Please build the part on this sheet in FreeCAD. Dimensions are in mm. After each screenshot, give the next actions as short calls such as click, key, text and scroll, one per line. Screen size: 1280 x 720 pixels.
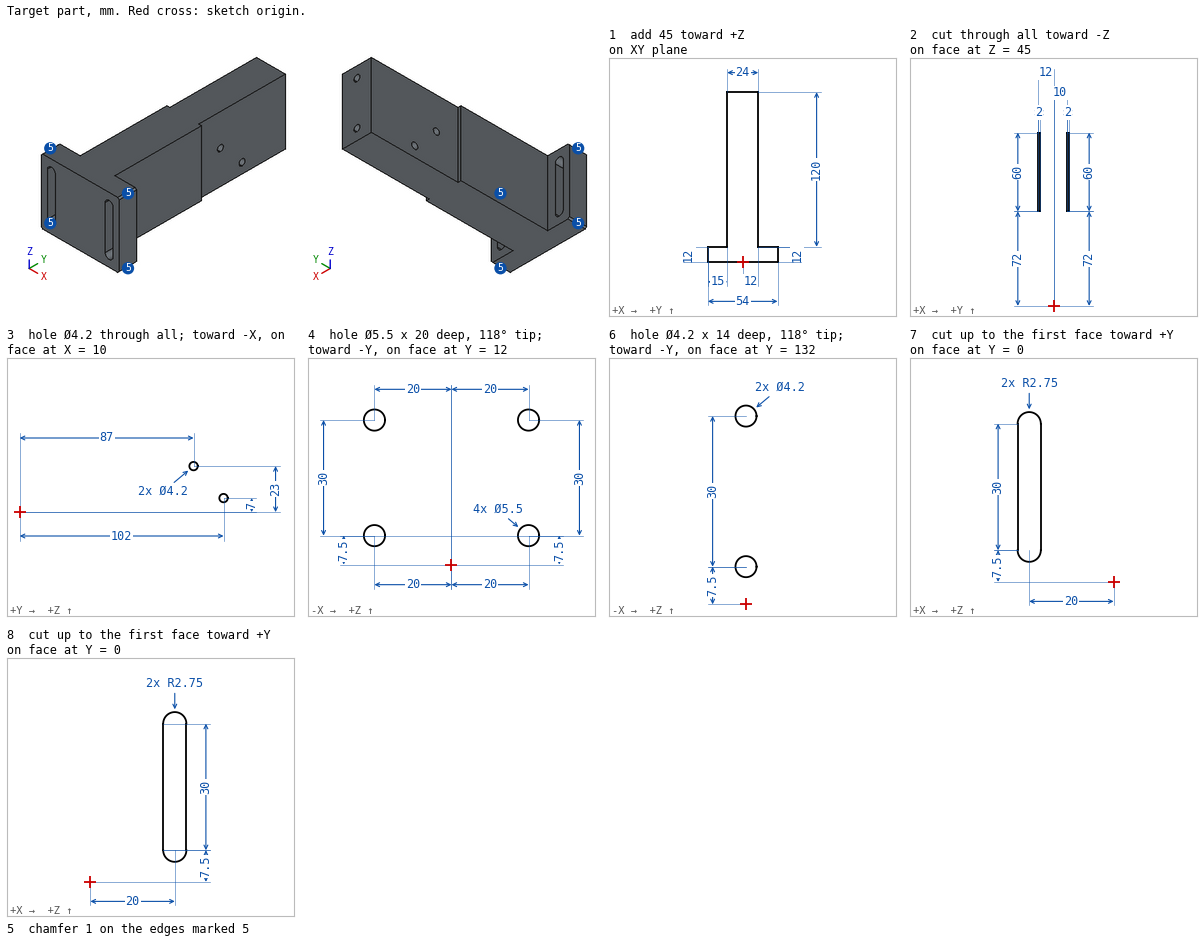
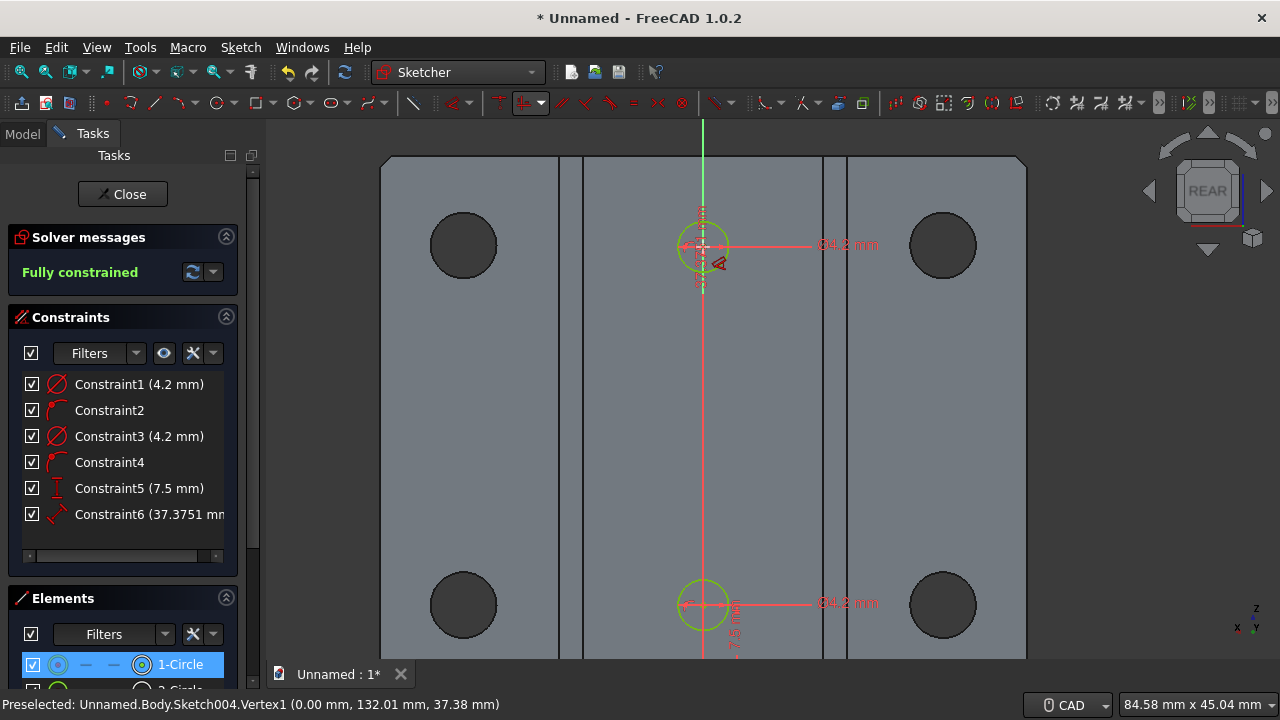
click(703, 605)
click(737, 426)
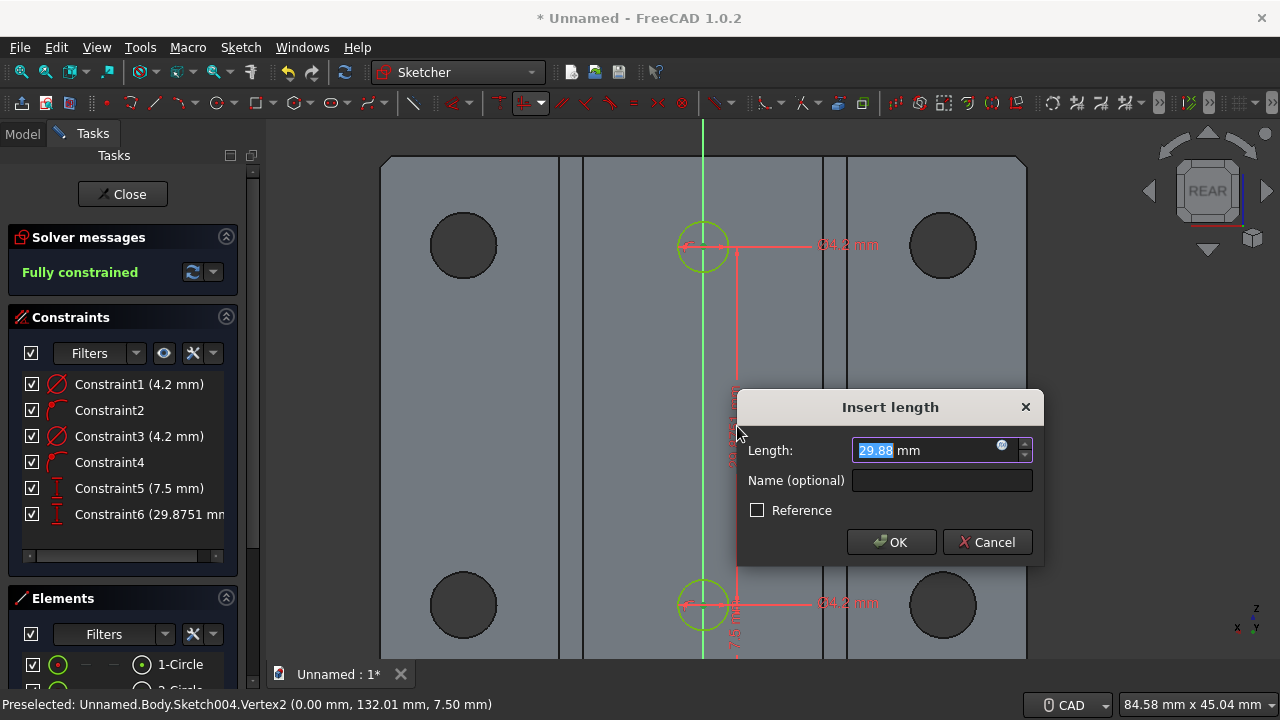
text(30)
key(Return)
key(Escape)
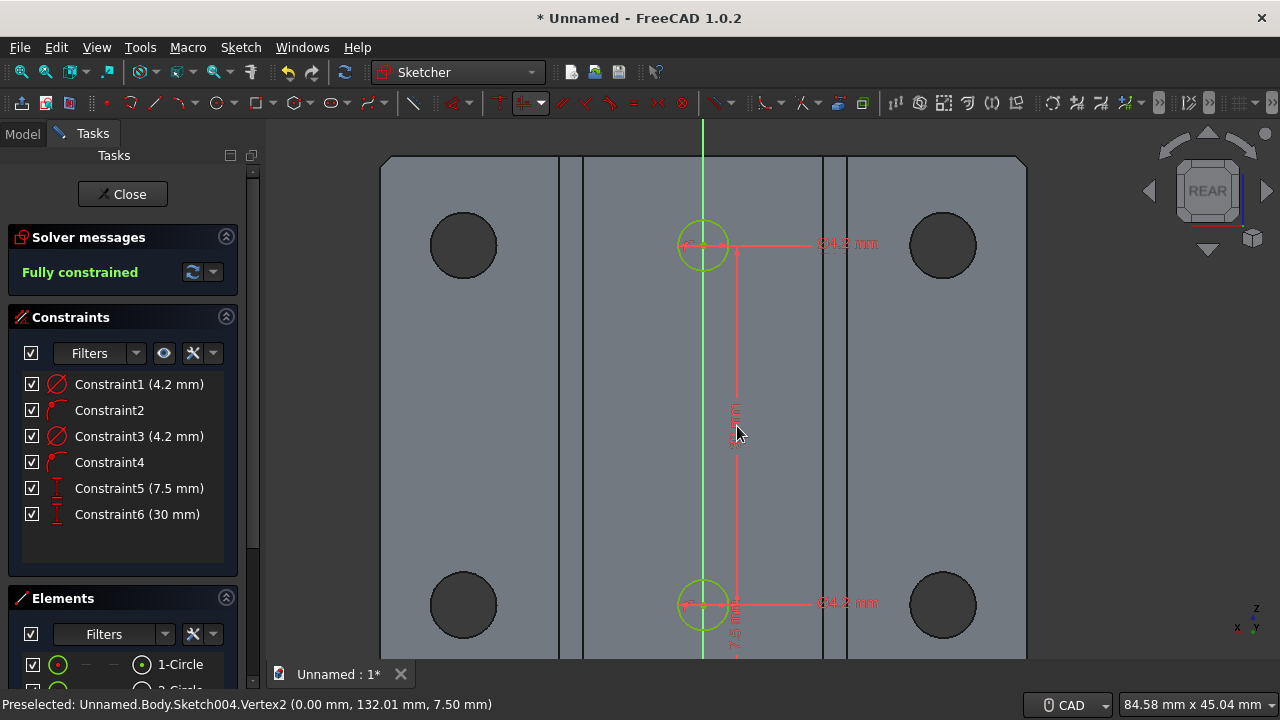
click(123, 194)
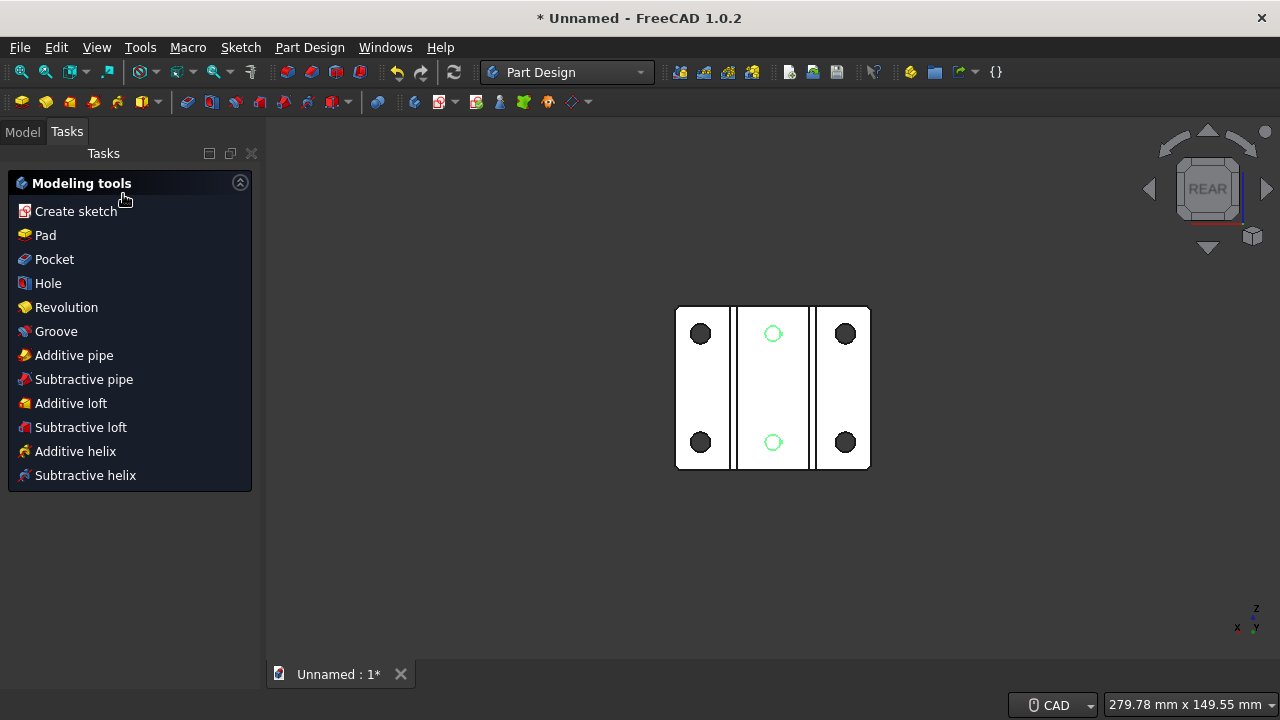
click(212, 102)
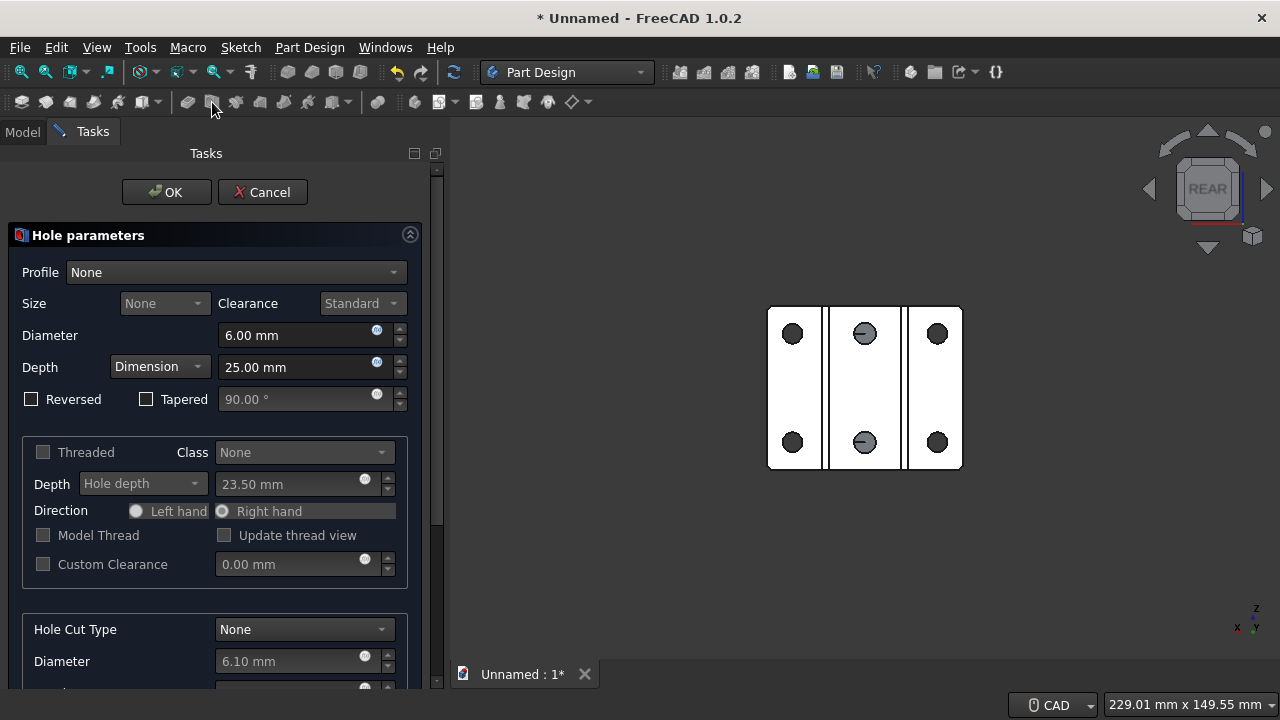
triple_click(305, 335)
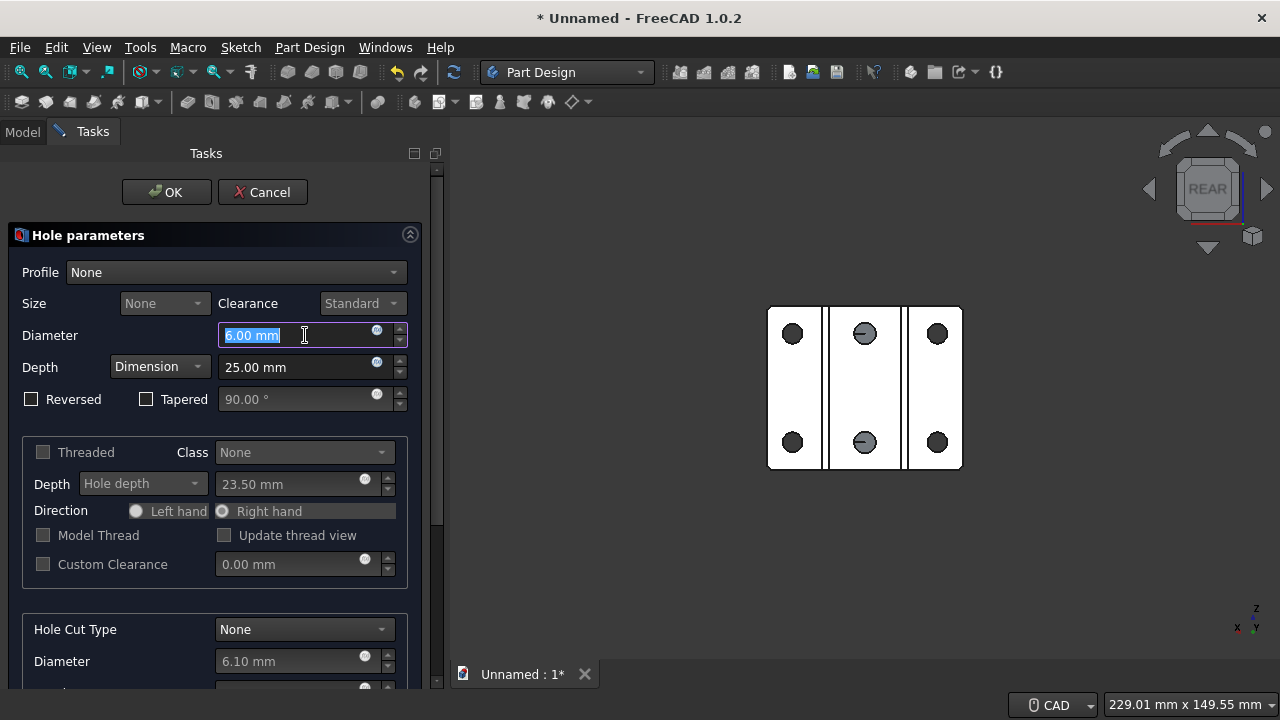
text(4.2)
key(Tab)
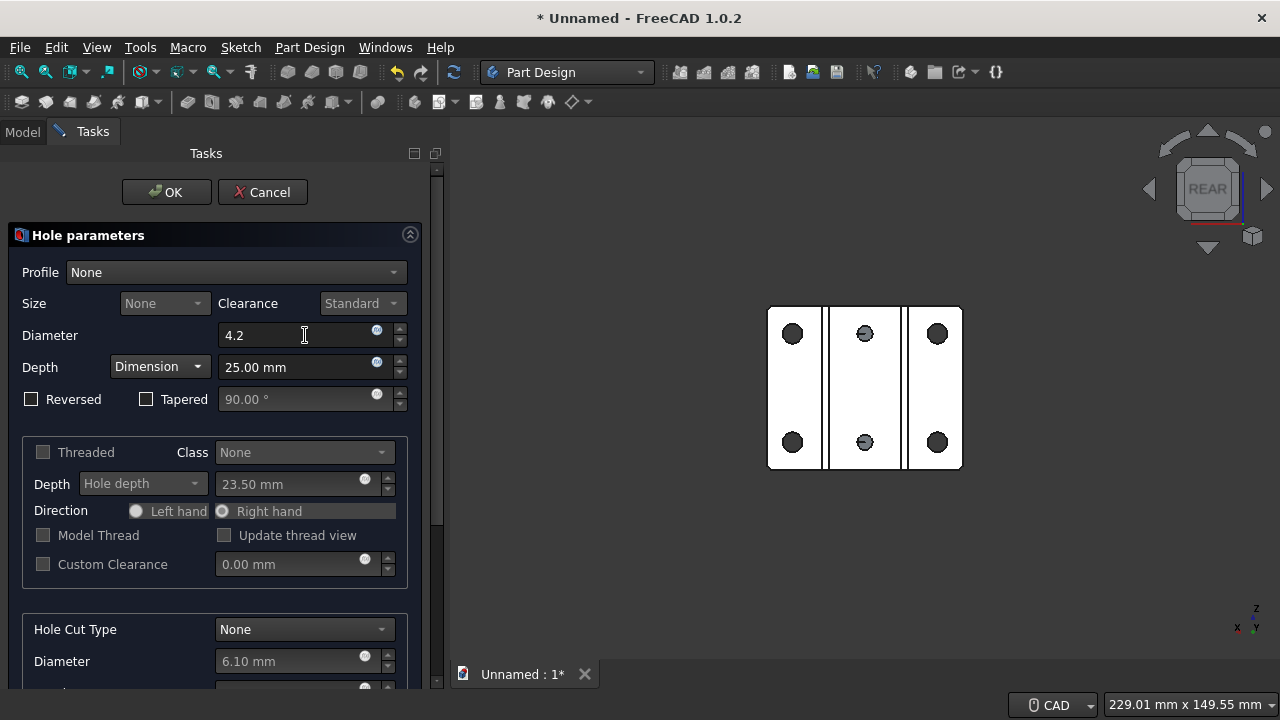
triple_click(305, 367)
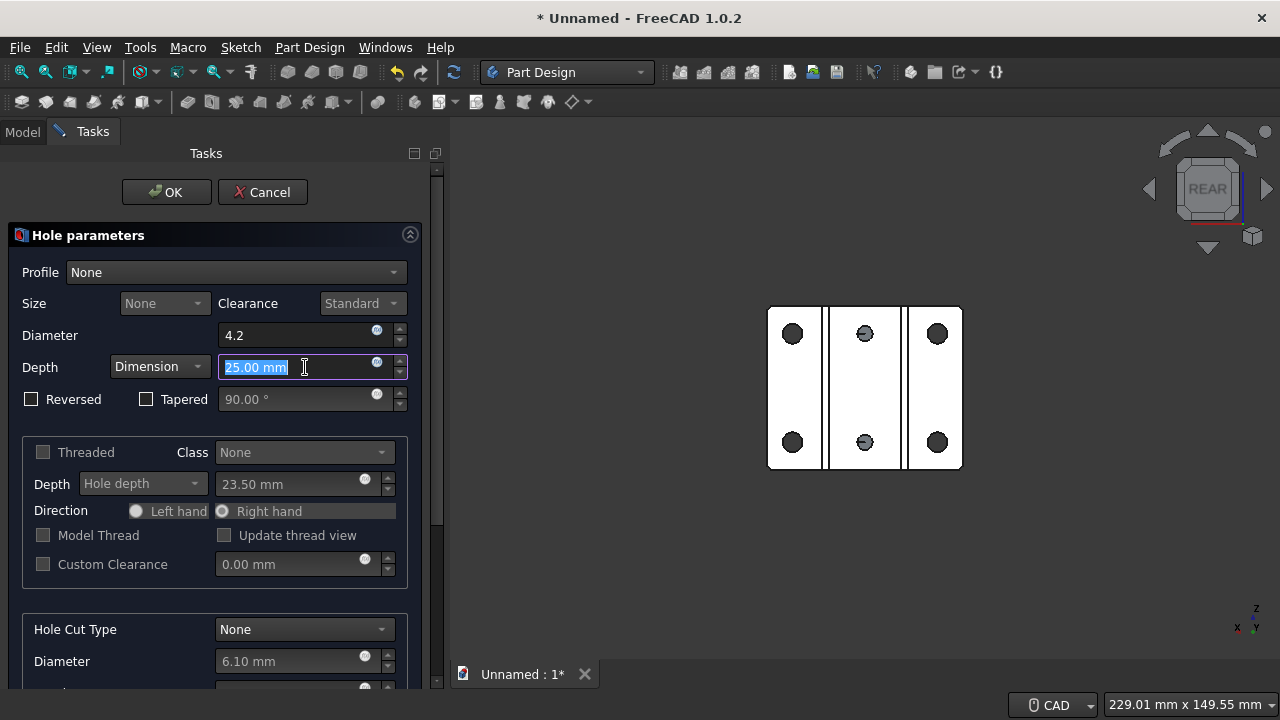
text(14)
key(Tab)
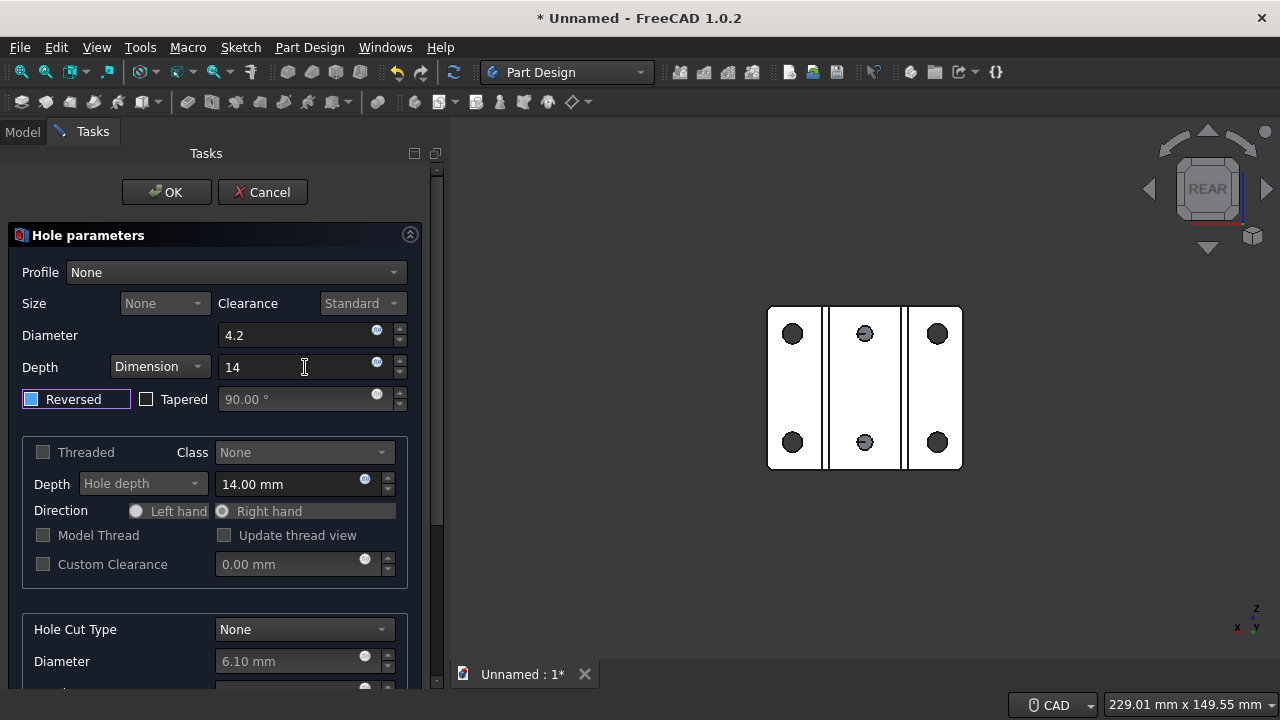
click(167, 192)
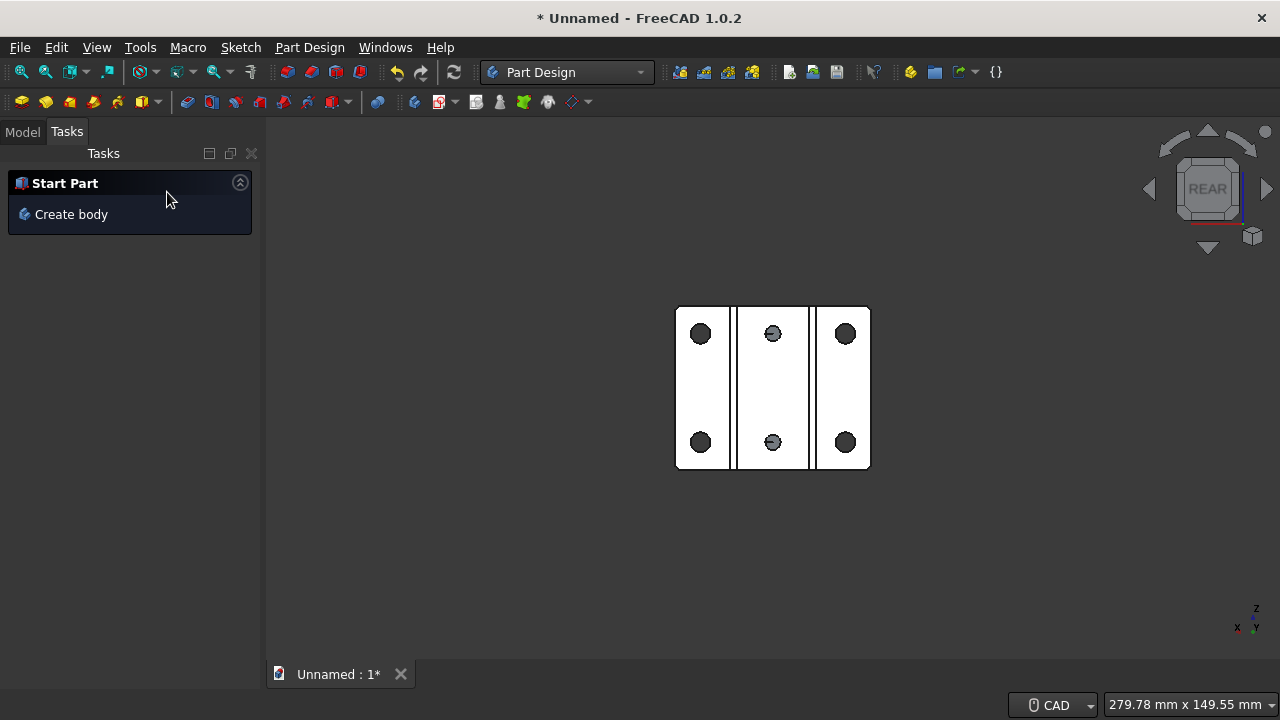
click(22, 72)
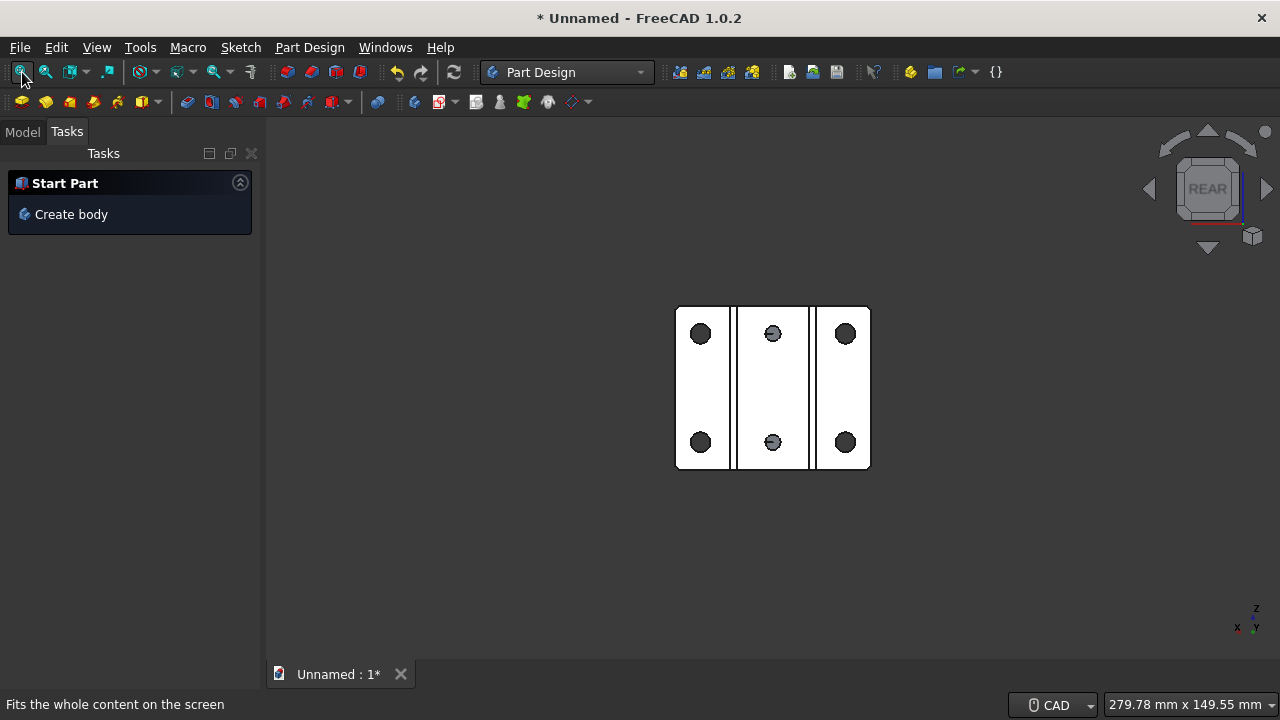
key(0)